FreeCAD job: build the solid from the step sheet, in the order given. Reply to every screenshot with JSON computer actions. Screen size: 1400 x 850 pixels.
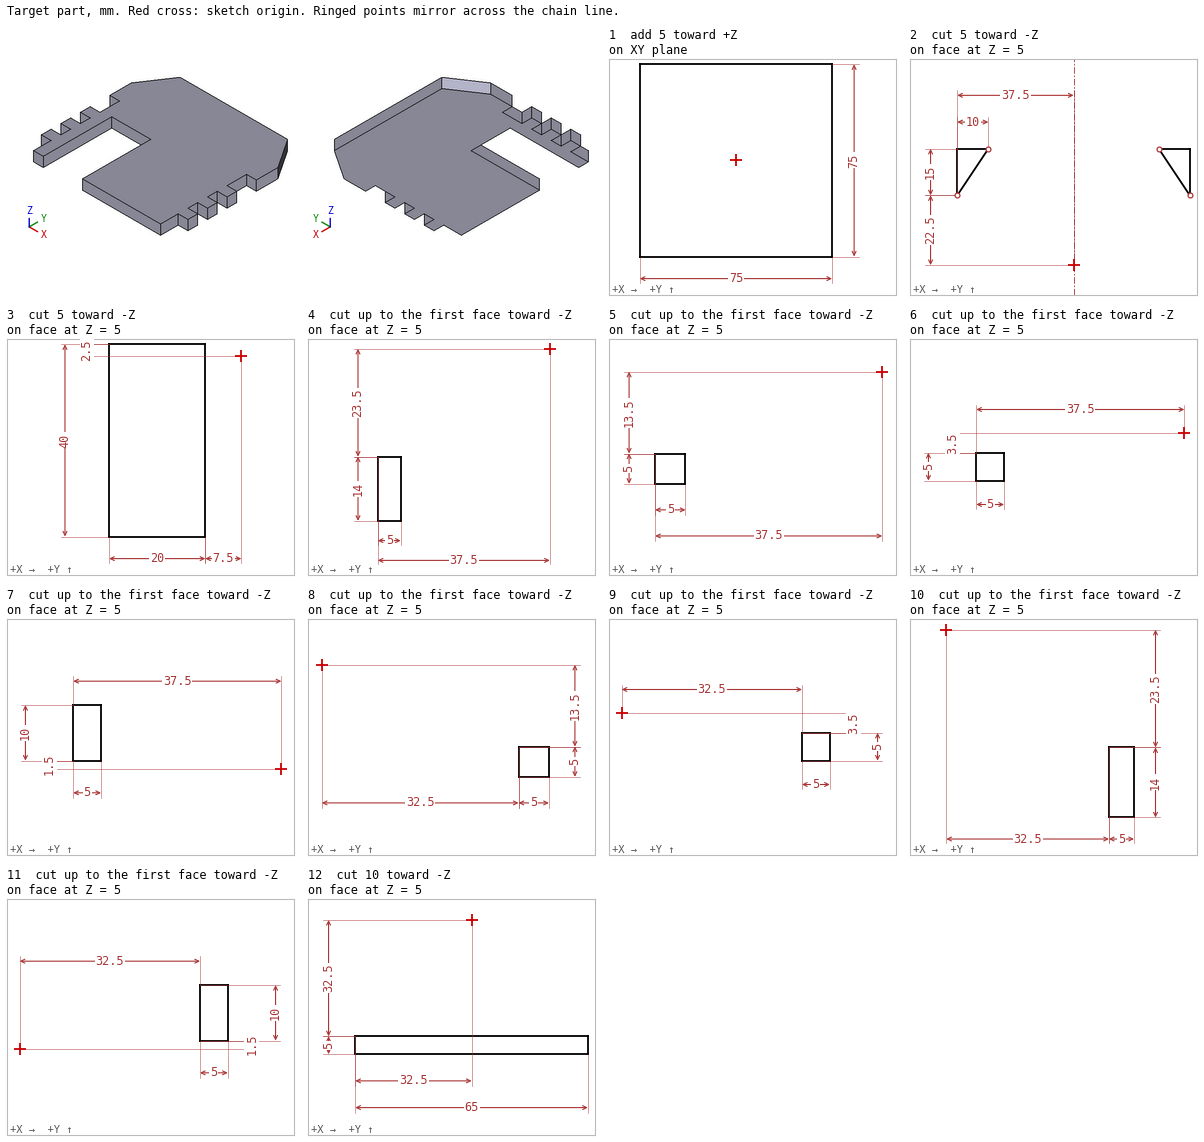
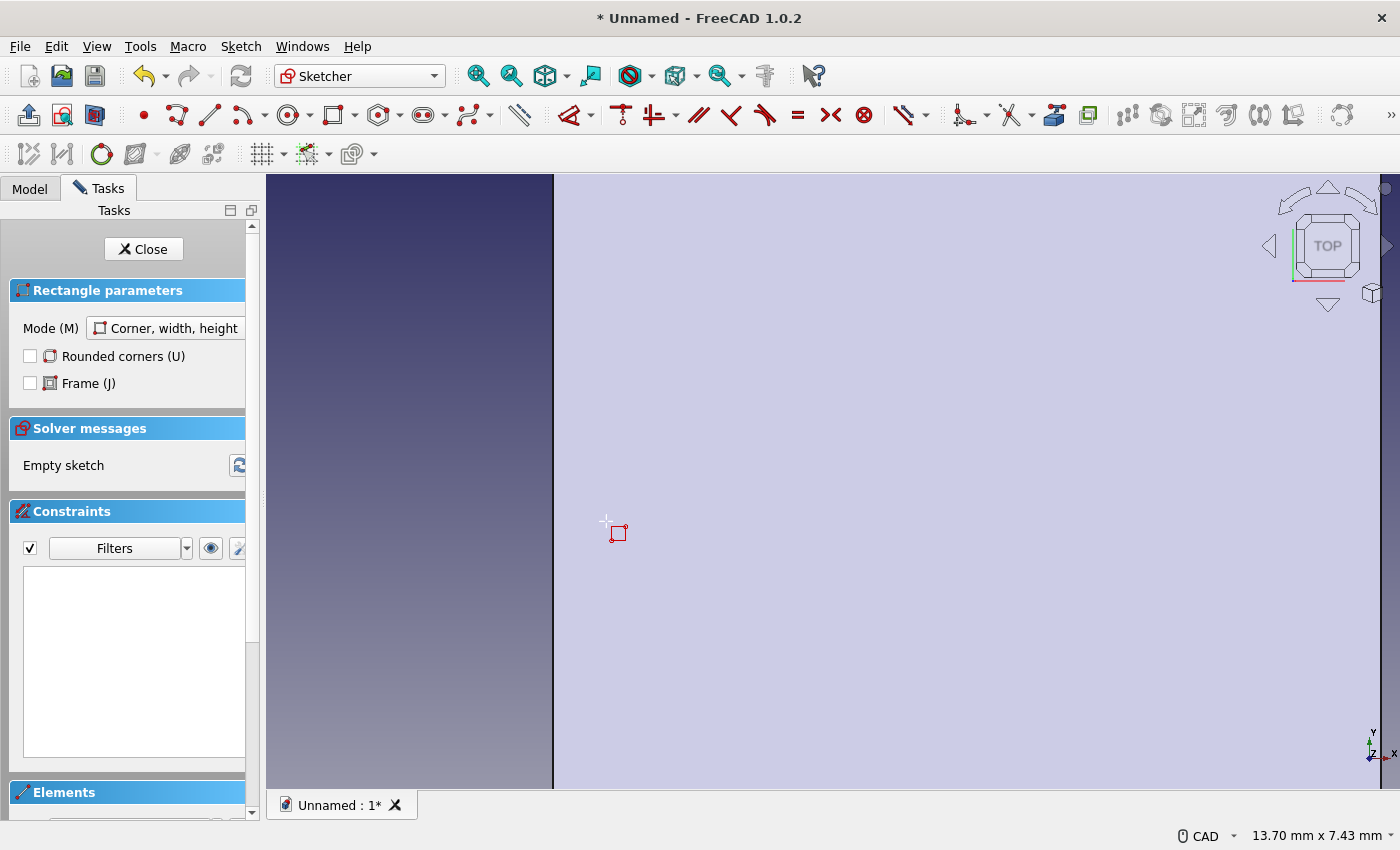
{"action": "left_click", "coordinate": [553, 272]}
{"action": "left_click", "coordinate": [967, 686]}
{"action": "key", "text": "Escape"}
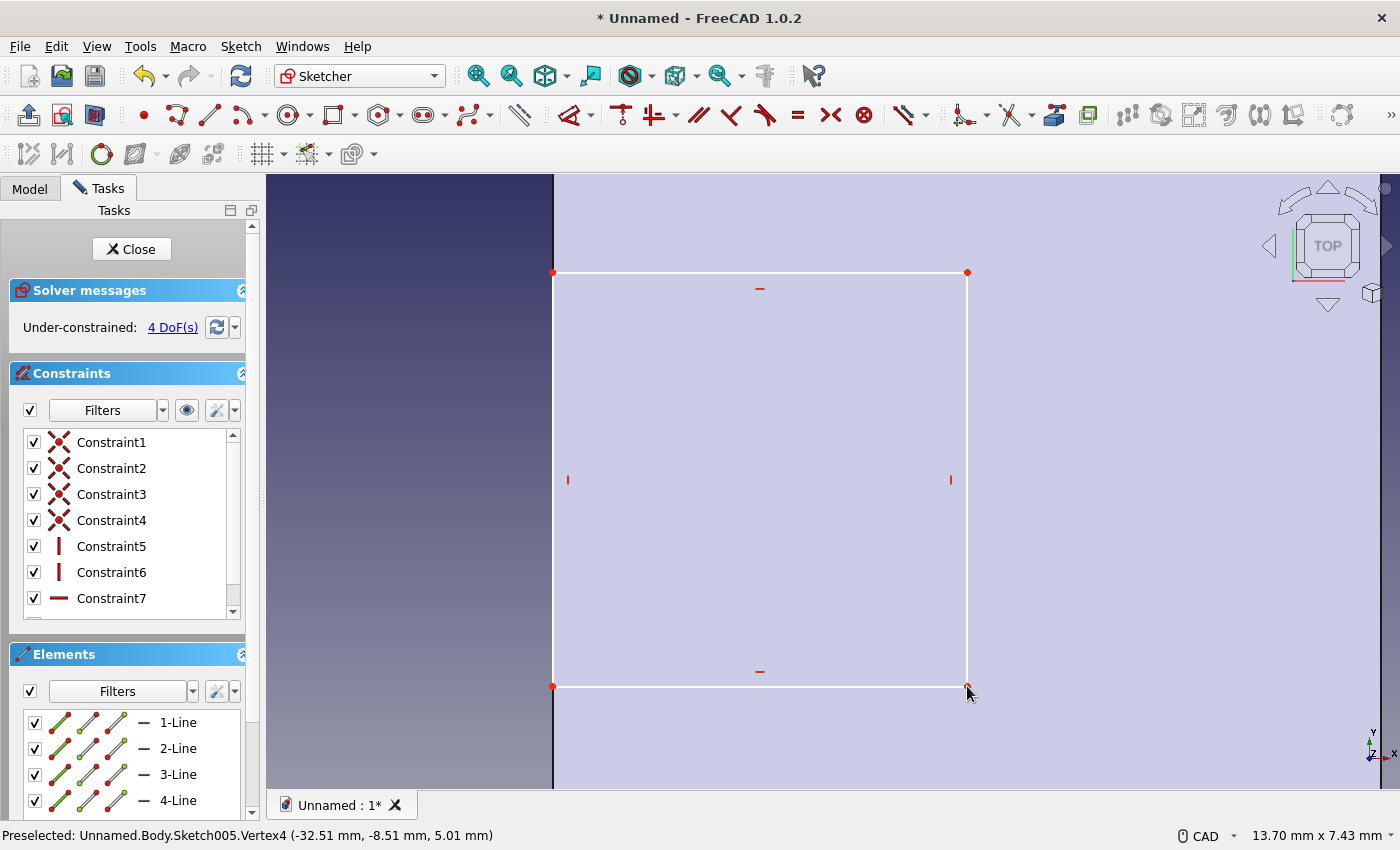
{"action": "left_click", "coordinate": [568, 116]}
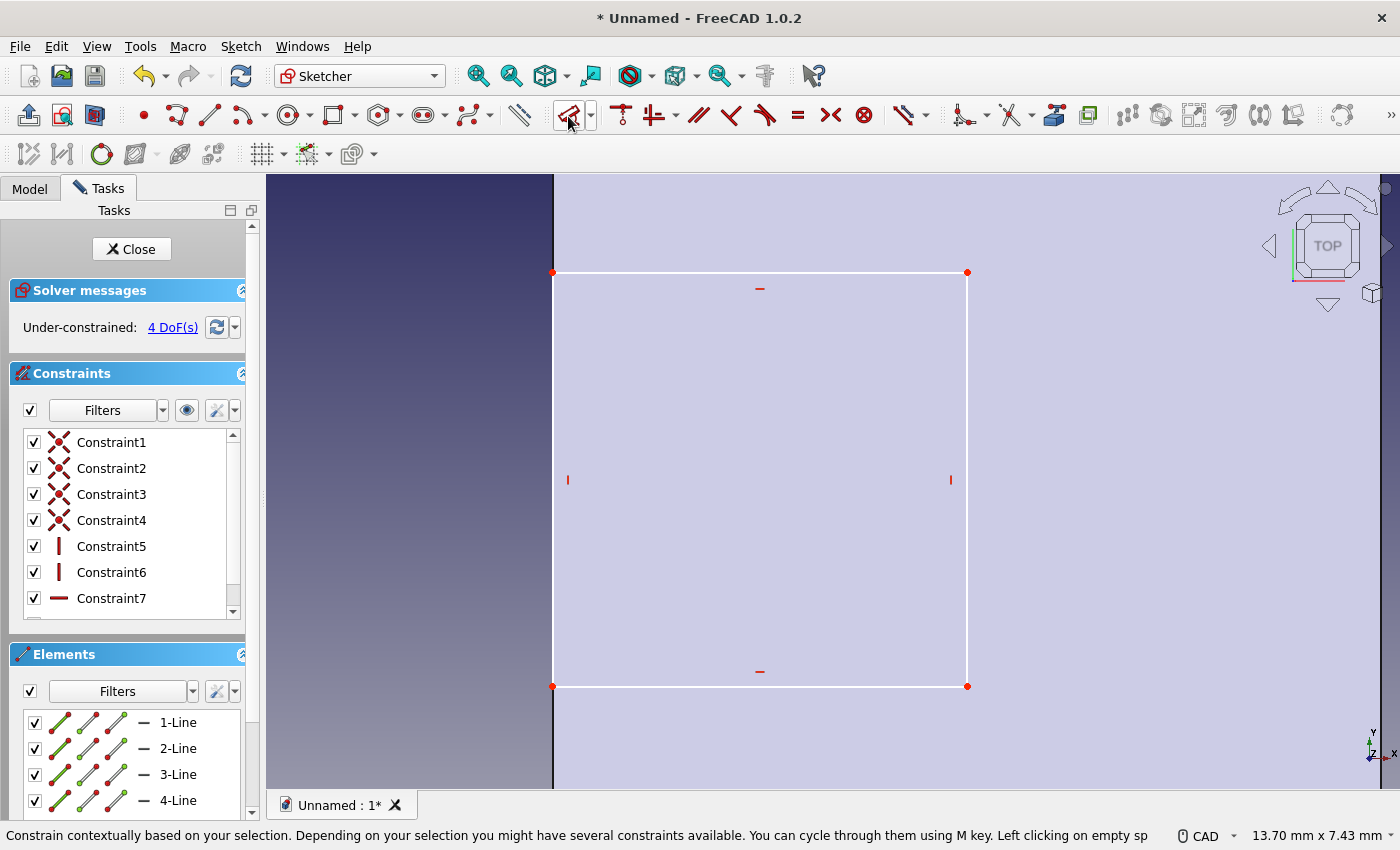
{"action": "left_click", "coordinate": [553, 397]}
{"action": "left_click", "coordinate": [519, 480]}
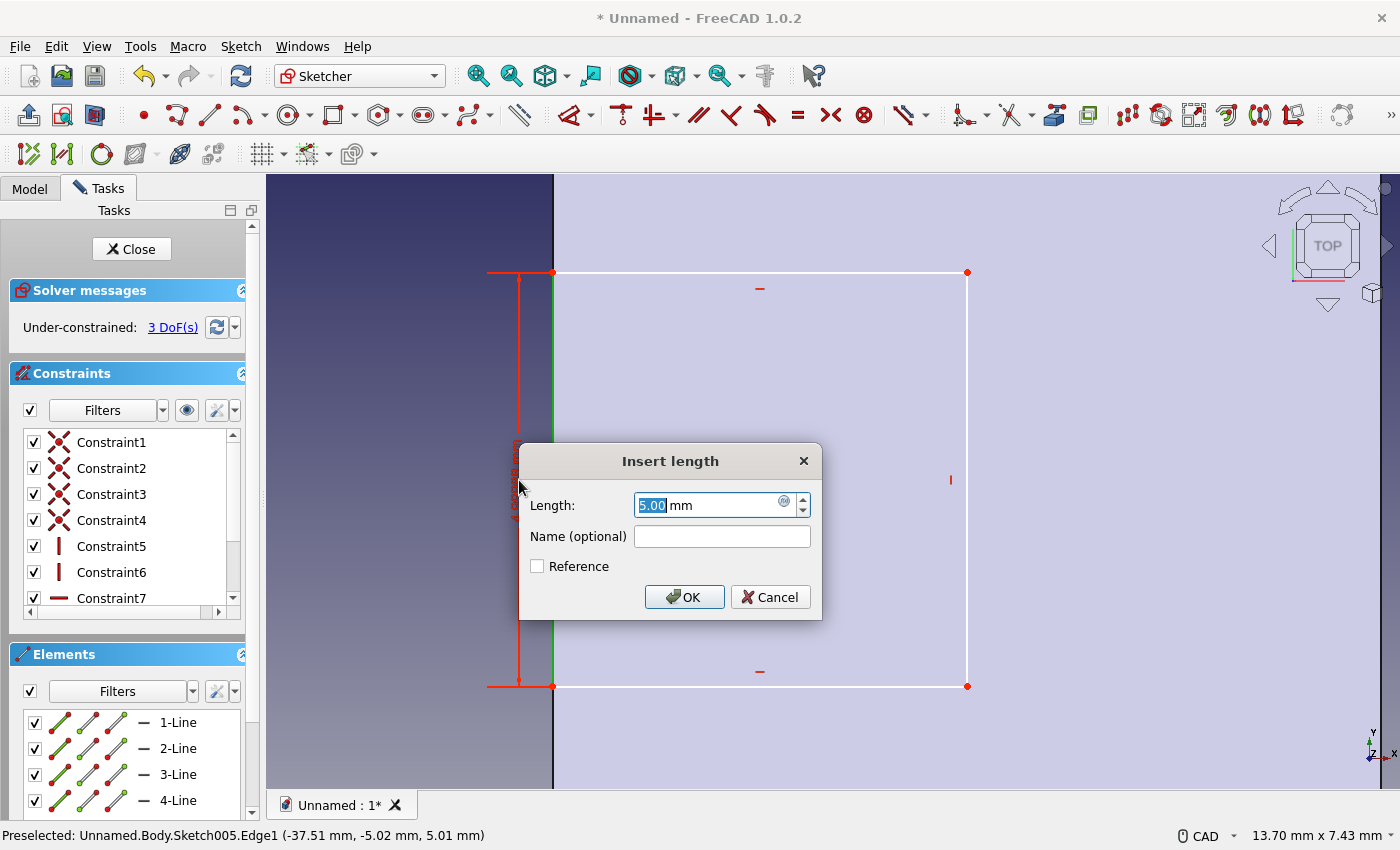
{"action": "type", "text": "5"}
{"action": "key", "text": "Return"}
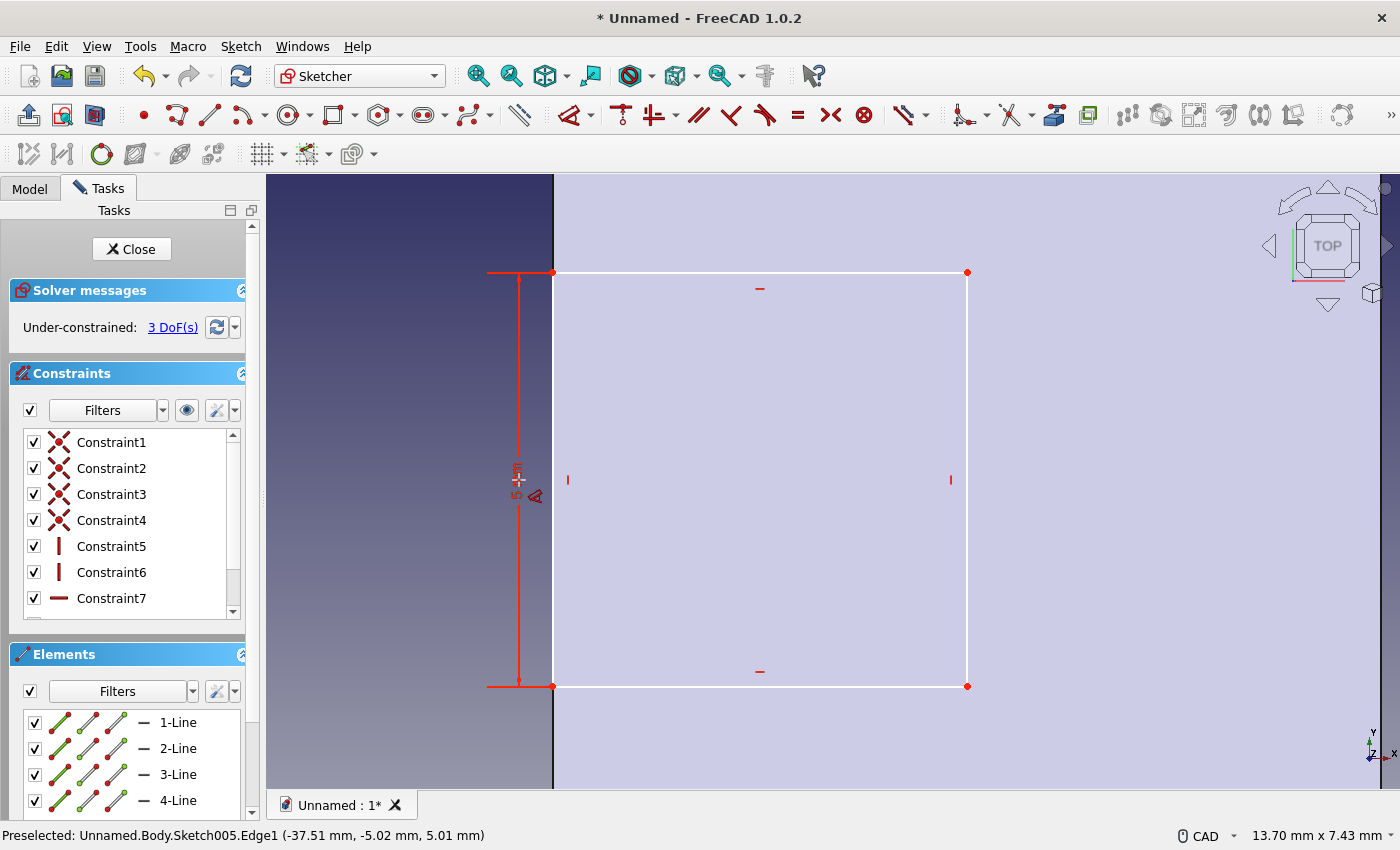
{"action": "left_click", "coordinate": [677, 687]}
{"action": "left_click", "coordinate": [760, 721]}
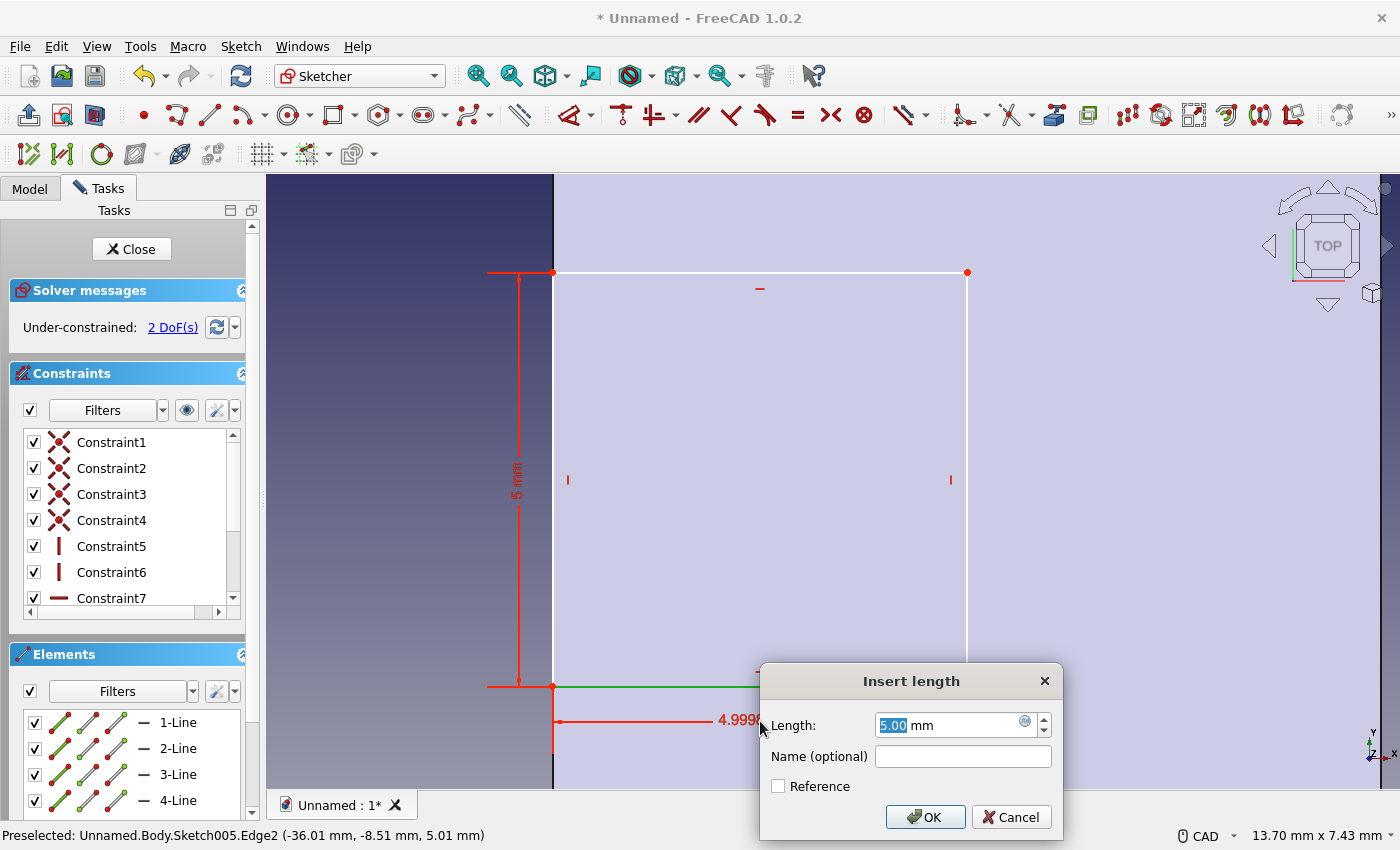
{"action": "type", "text": "5"}
{"action": "key", "text": "Return"}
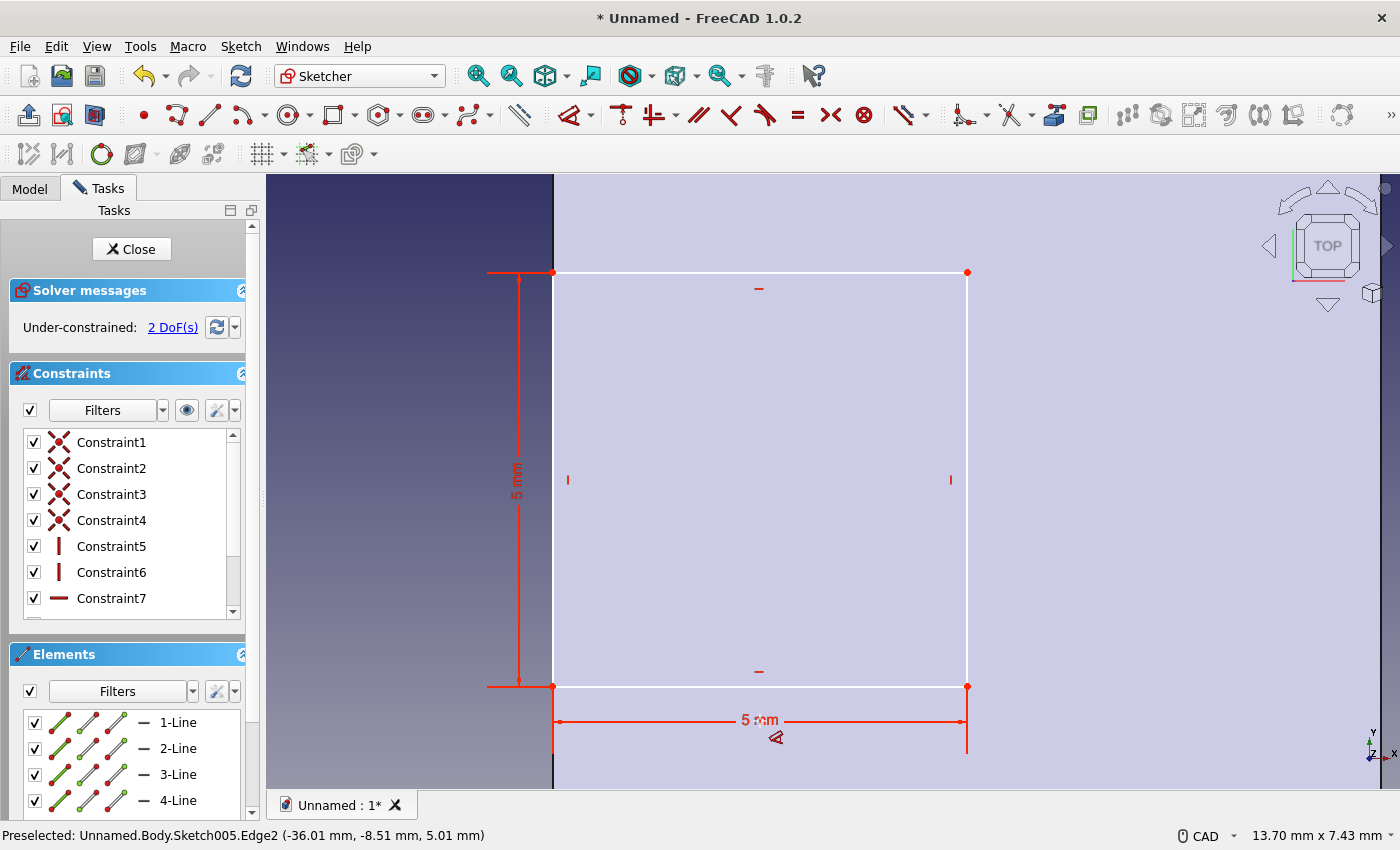
{"action": "left_click", "coordinate": [553, 273]}
{"action": "left_click", "coordinate": [519, 237]}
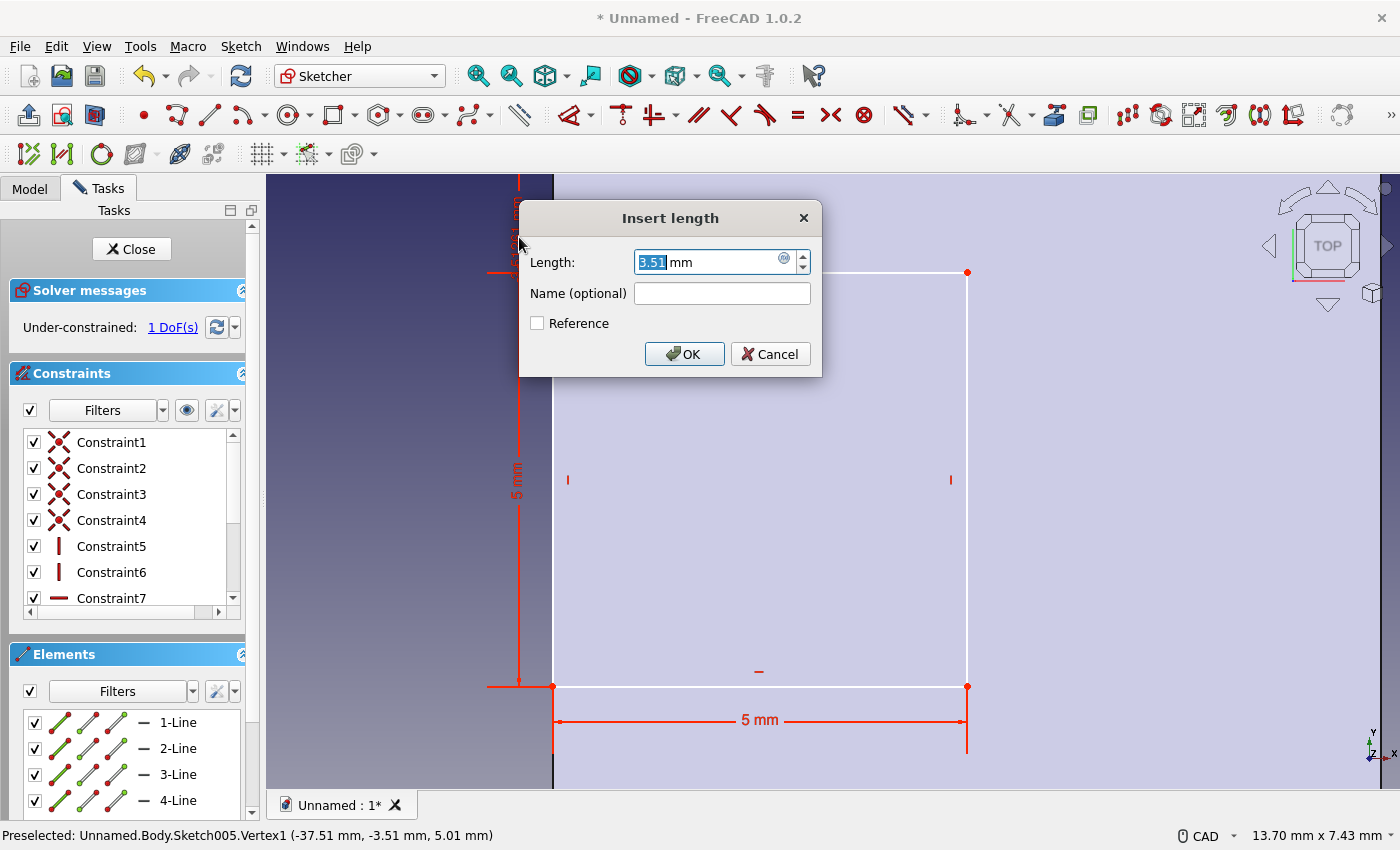
{"action": "type", "text": "3.5"}
{"action": "key", "text": "Return"}